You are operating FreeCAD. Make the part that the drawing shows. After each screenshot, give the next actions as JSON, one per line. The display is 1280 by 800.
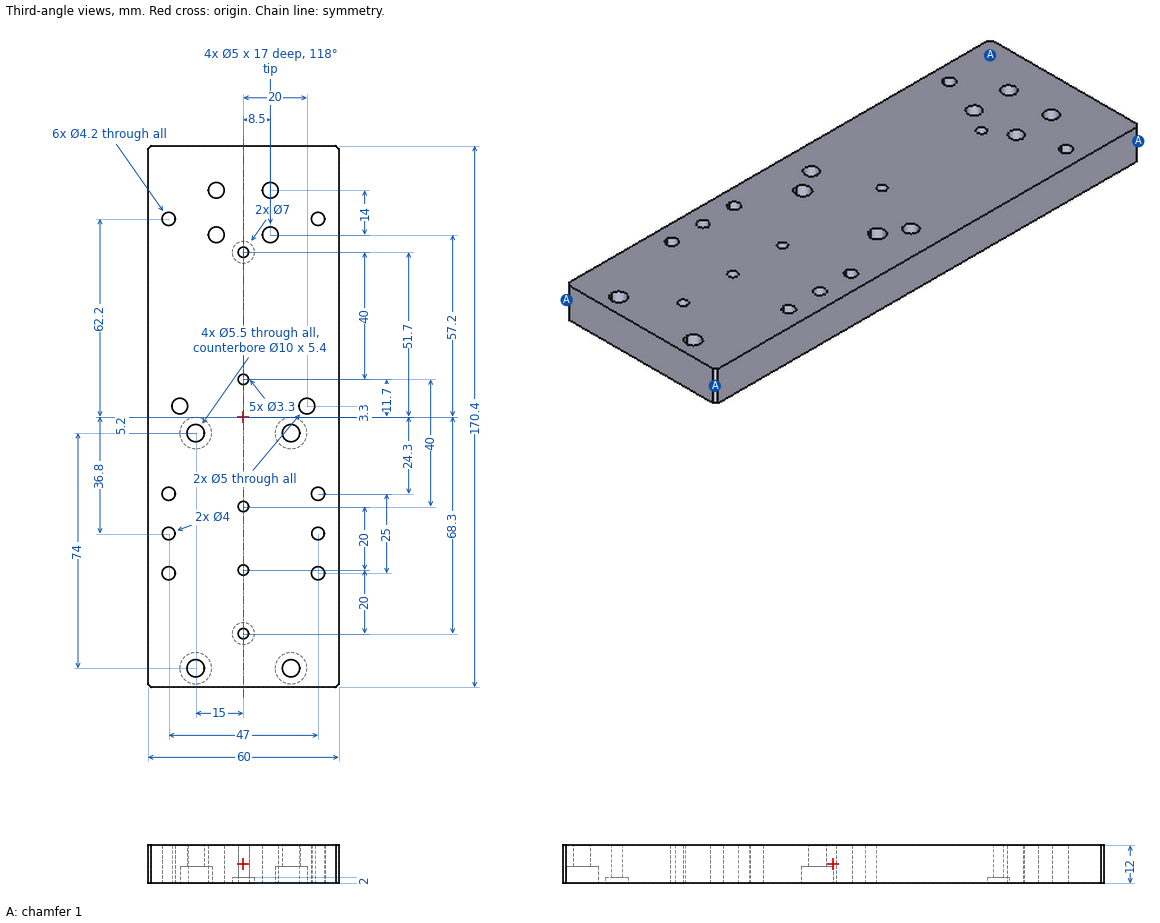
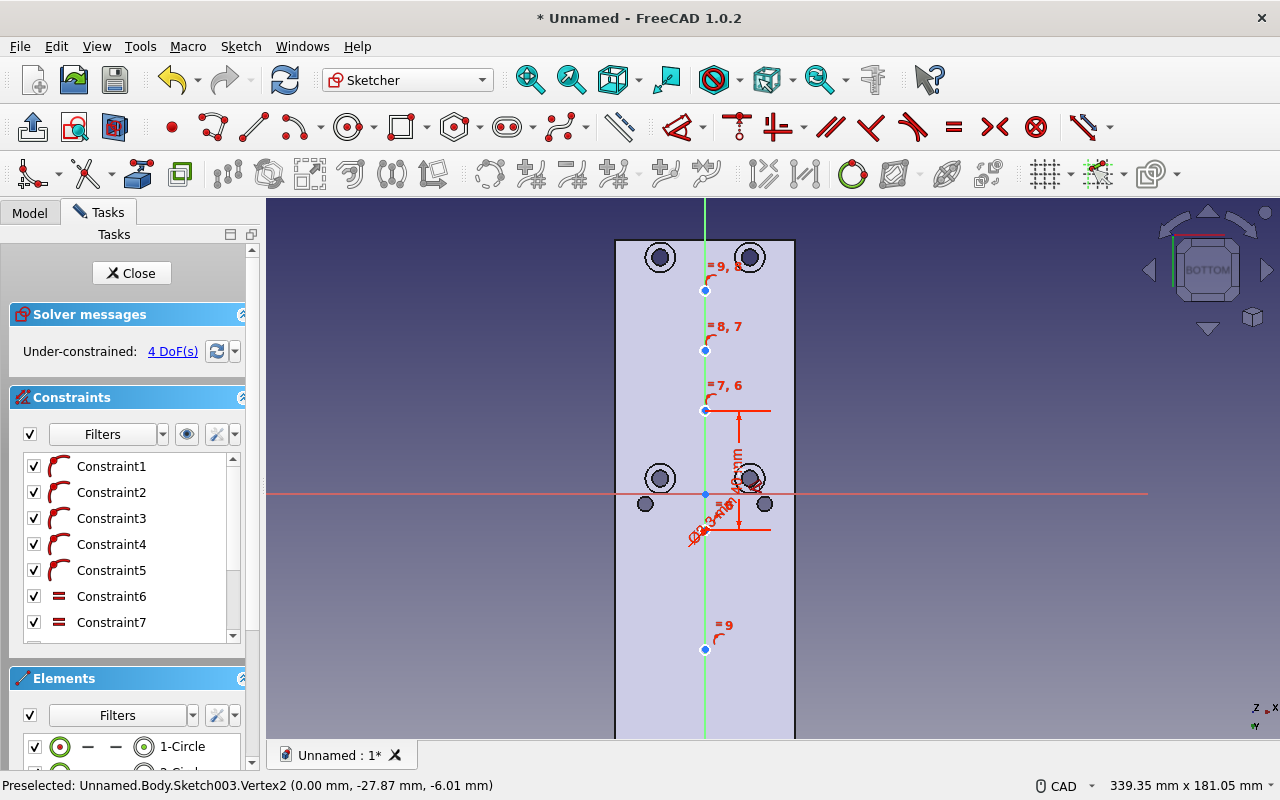
{"action": "left_click", "coordinate": [705, 411]}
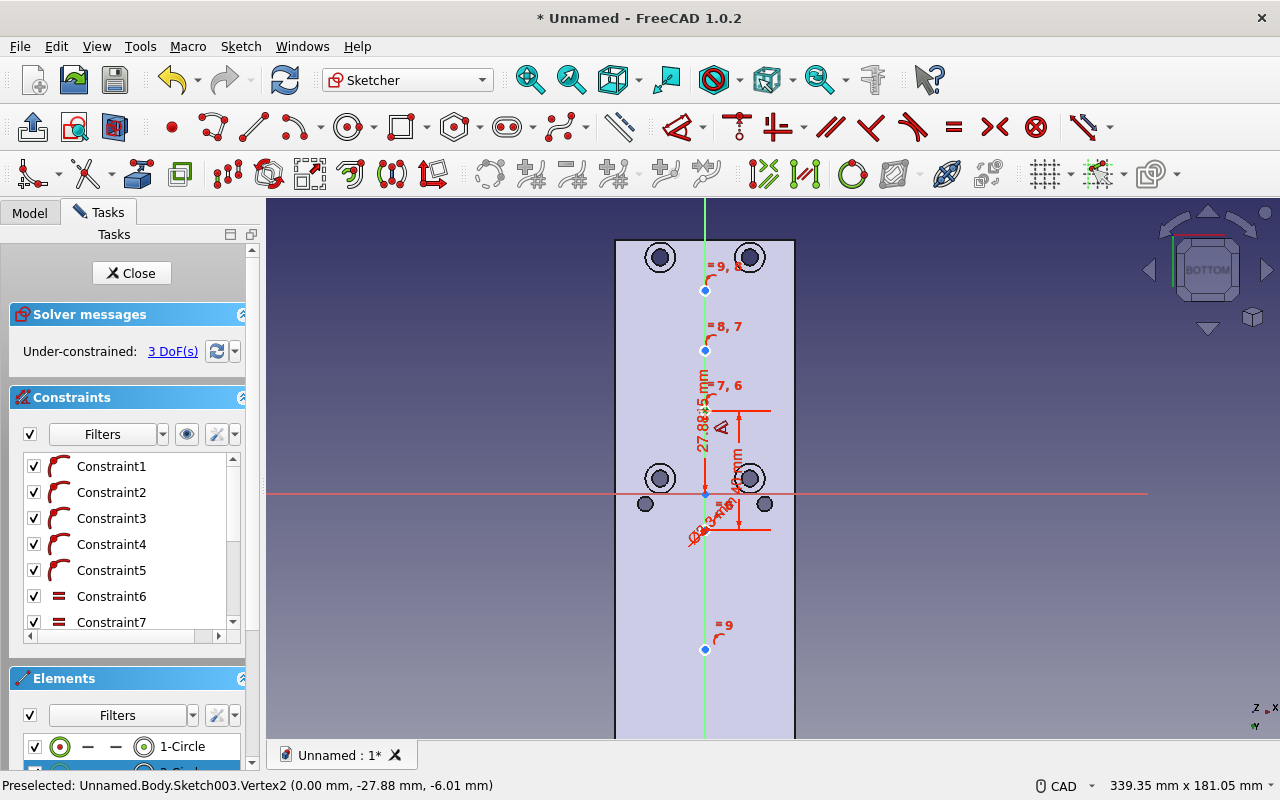
{"action": "left_click", "coordinate": [705, 351]}
{"action": "left_click", "coordinate": [739, 381]}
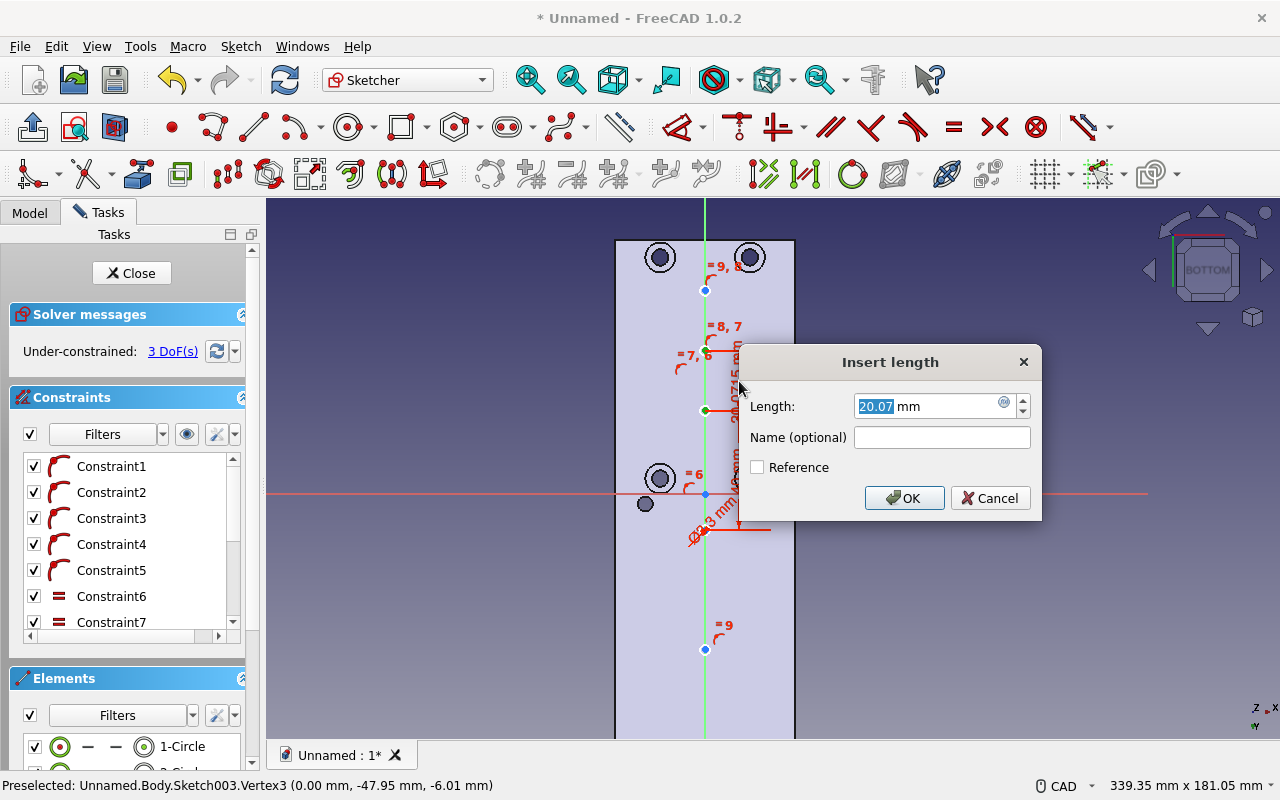
{"action": "type", "text": "20"}
{"action": "key", "text": "Return"}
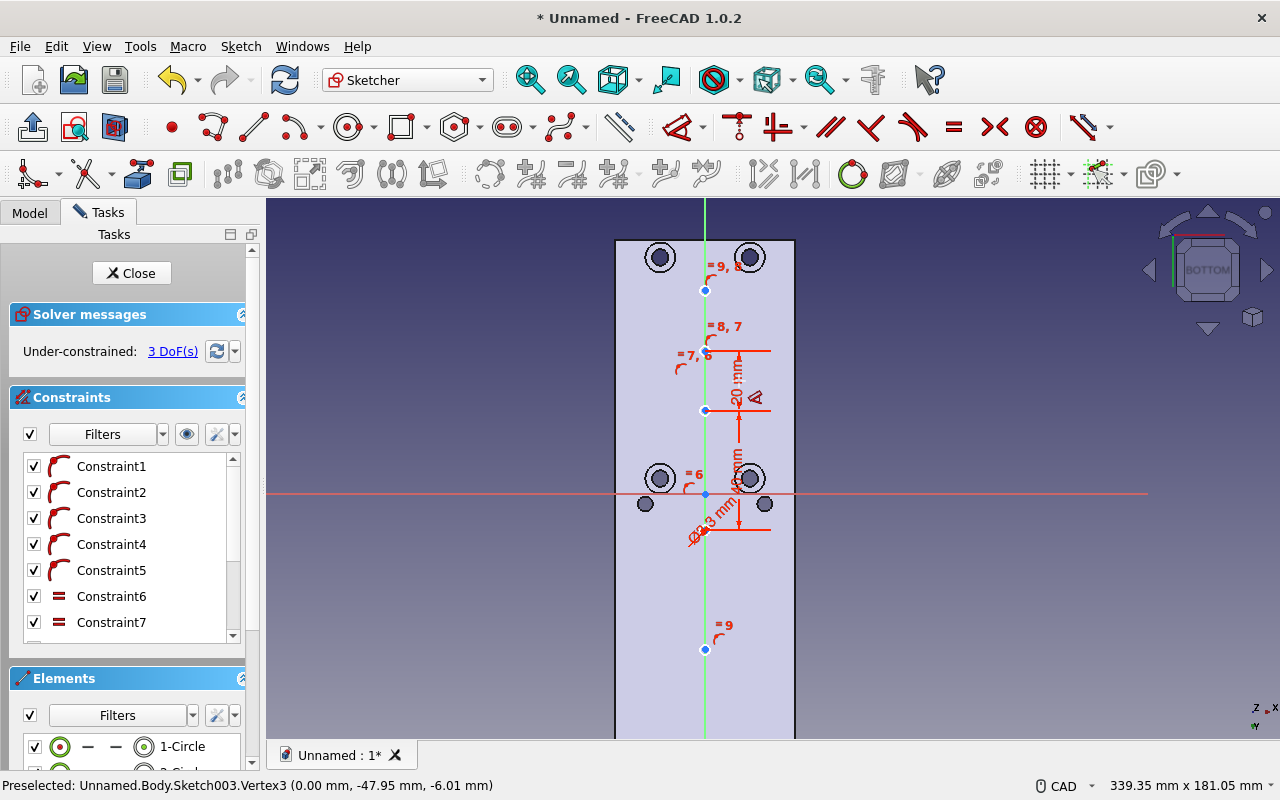
{"action": "left_click", "coordinate": [705, 351]}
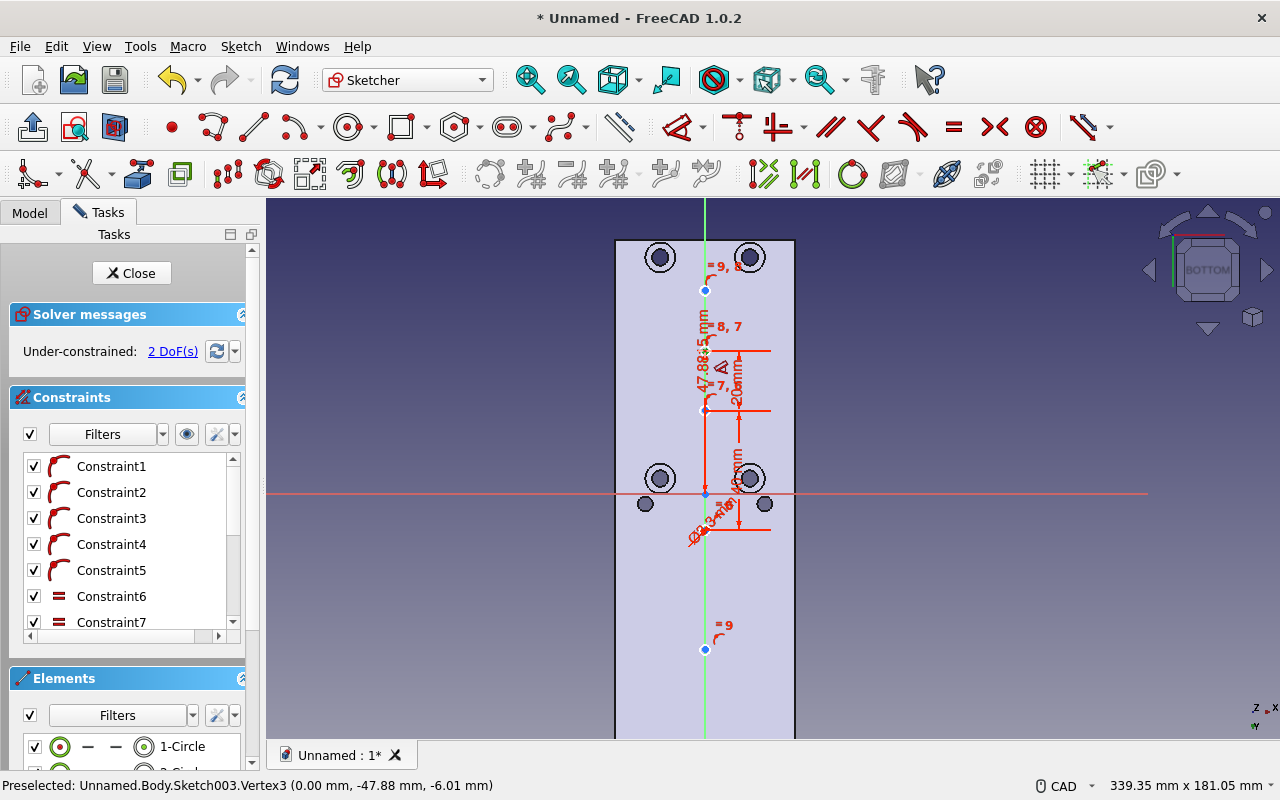
{"action": "left_click", "coordinate": [705, 291]}
{"action": "left_click", "coordinate": [739, 321]}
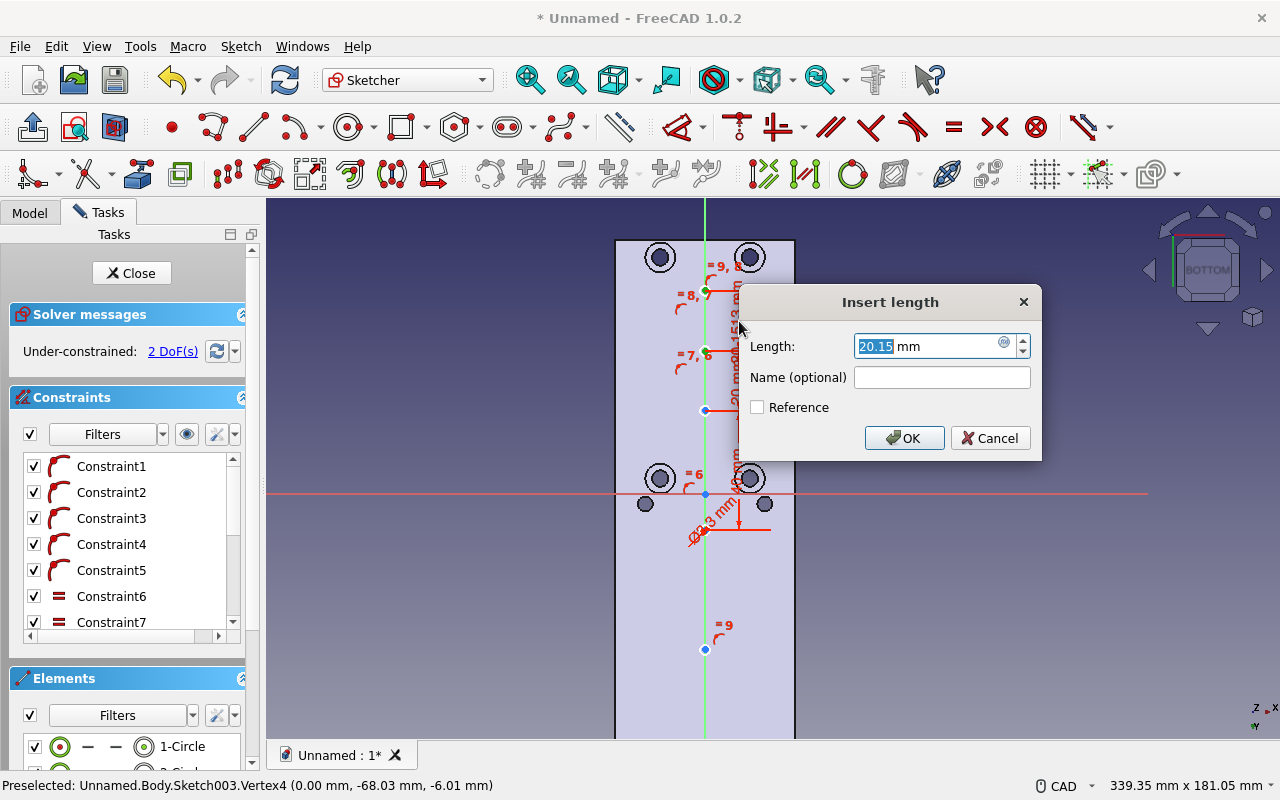
{"action": "type", "text": "20"}
{"action": "key", "text": "Return"}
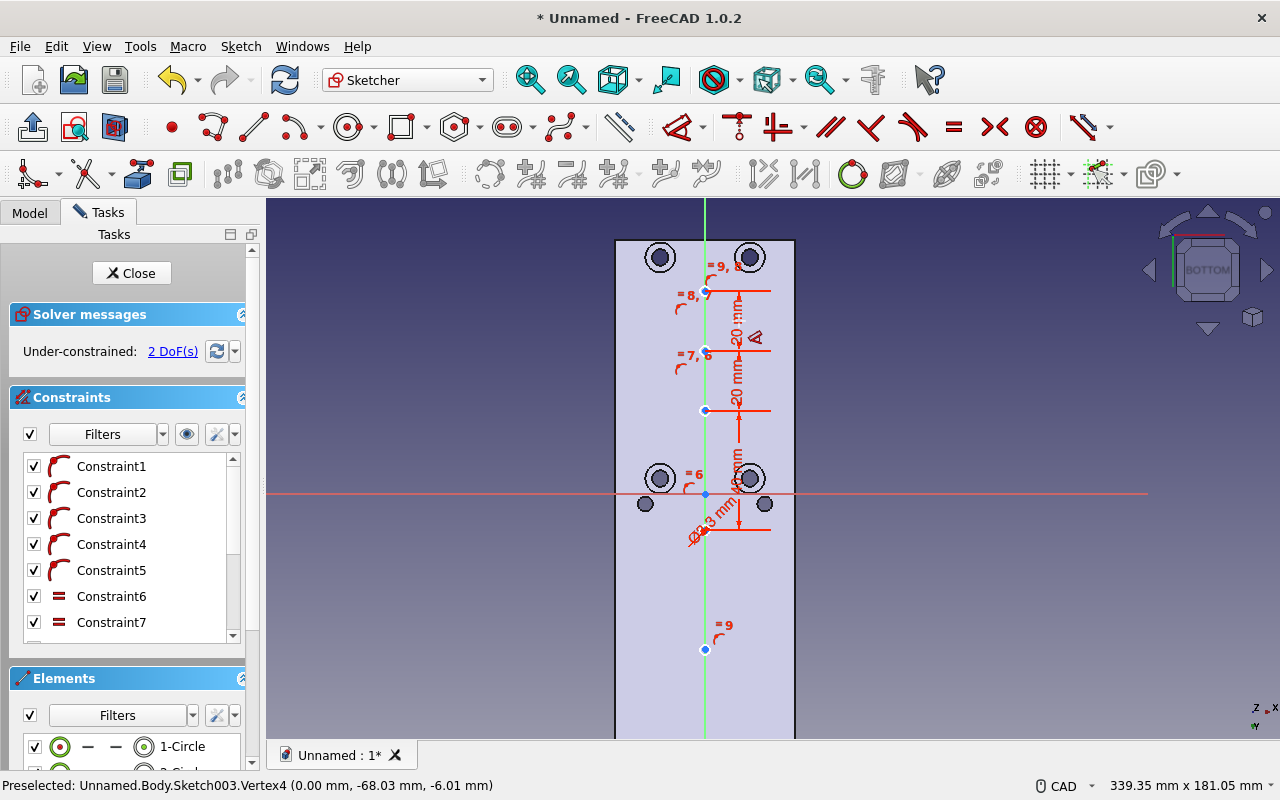
{"action": "left_click", "coordinate": [705, 530]}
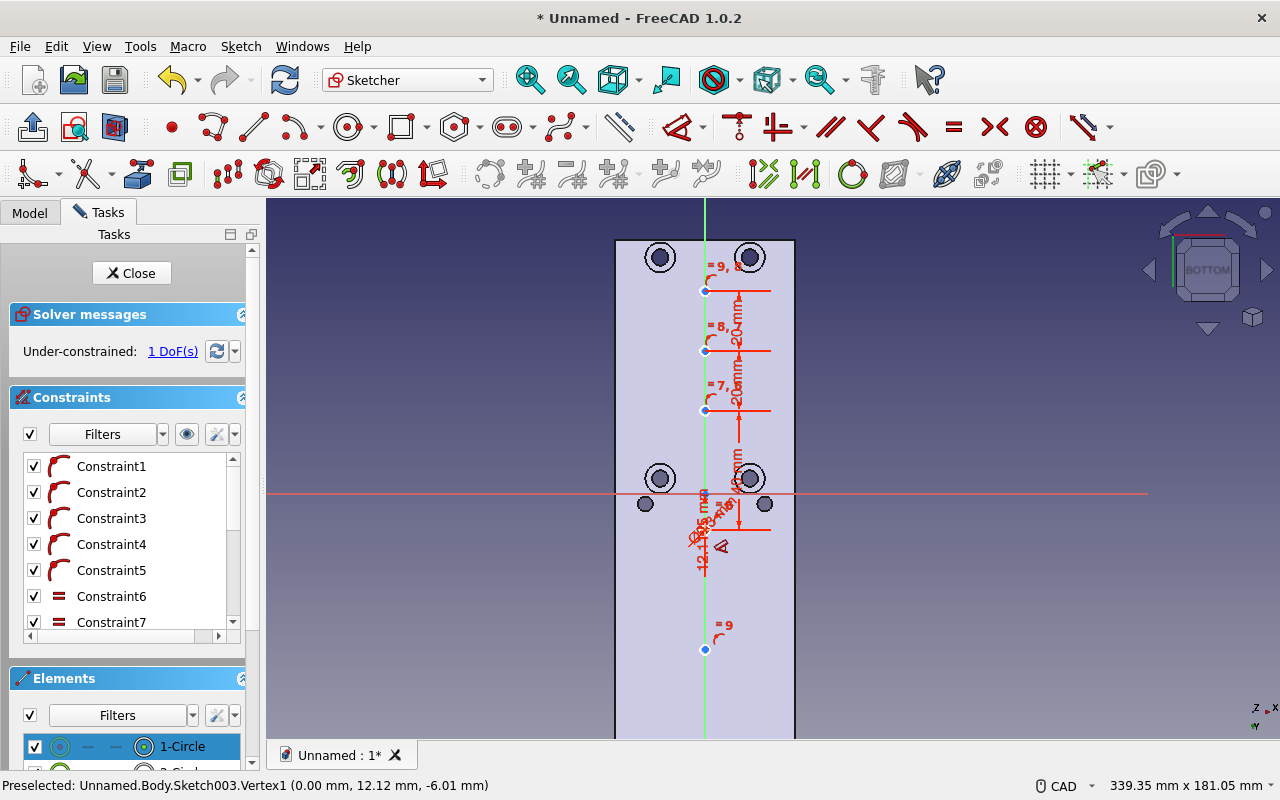
{"action": "left_click", "coordinate": [705, 650]}
{"action": "left_click", "coordinate": [739, 590]}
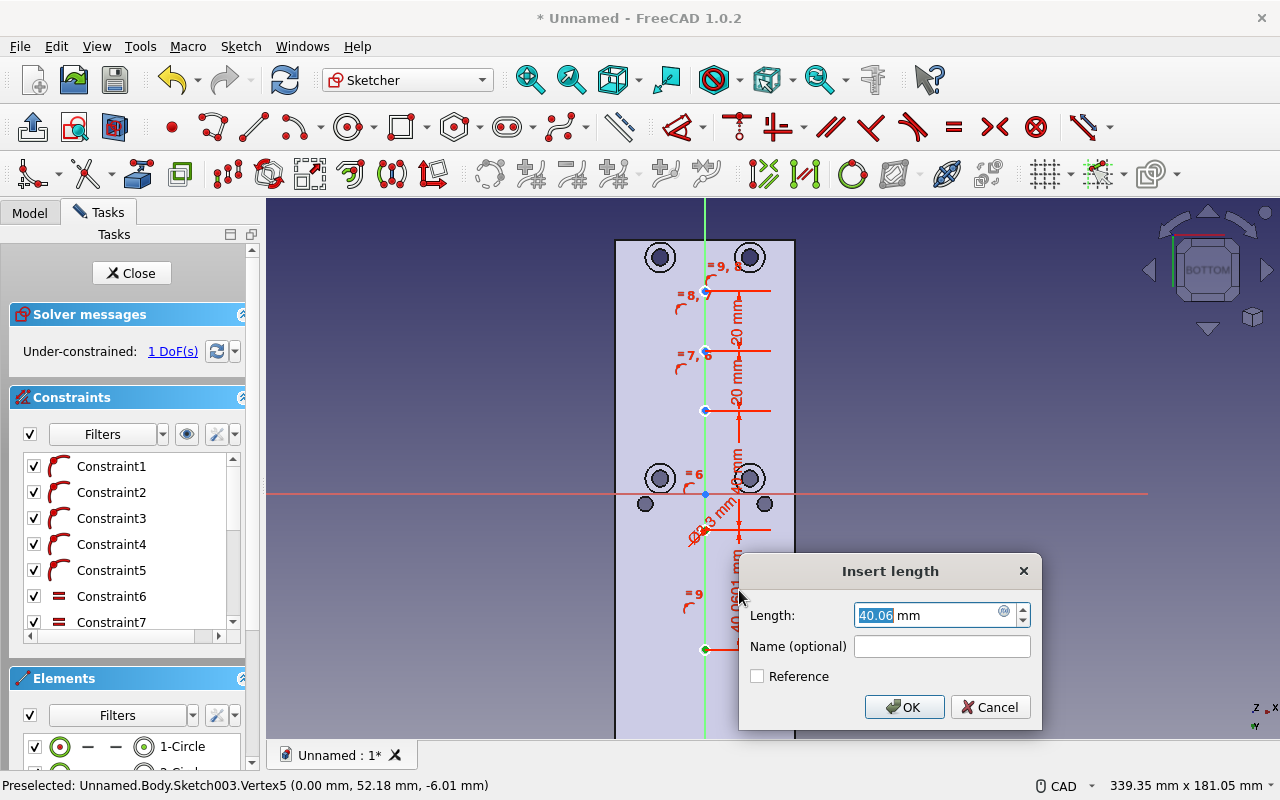
{"action": "type", "text": "40"}
{"action": "key", "text": "Return"}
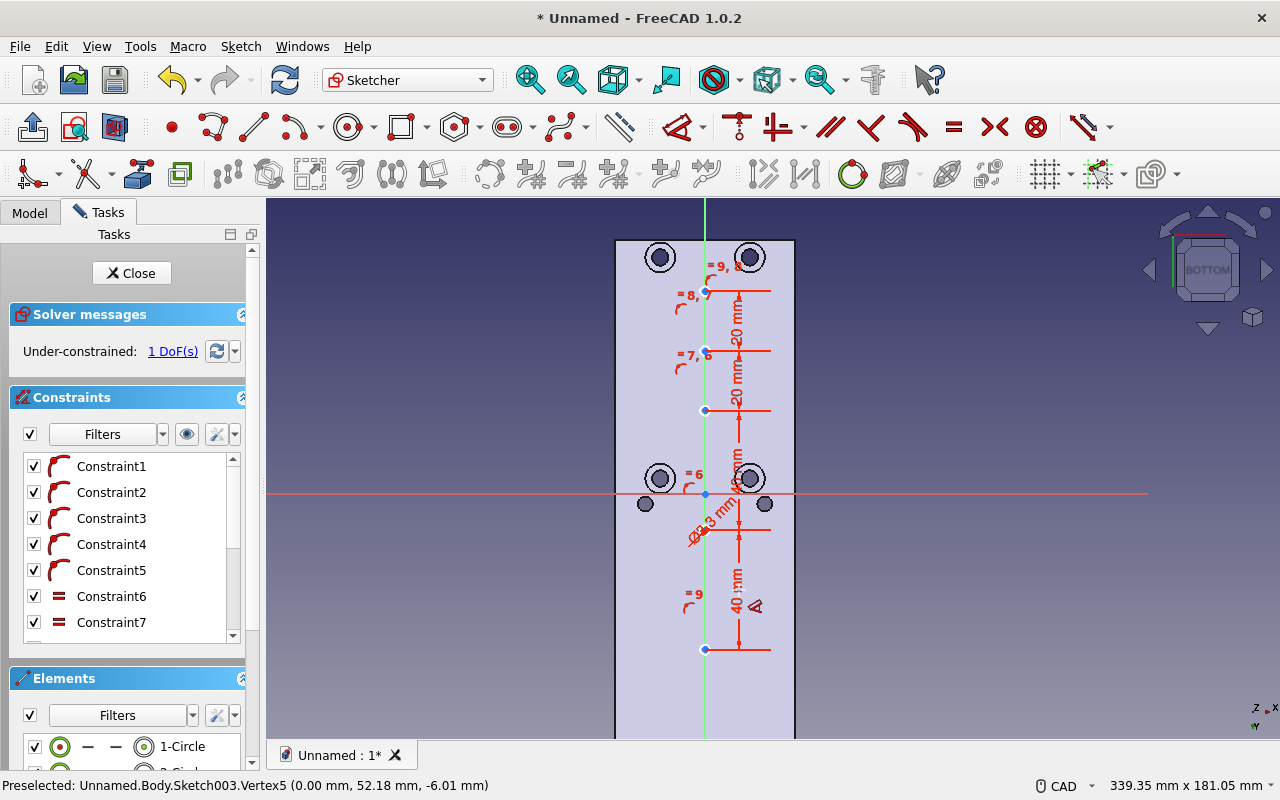
{"action": "left_click", "coordinate": [705, 530]}
{"action": "left_click", "coordinate": [787, 512]}